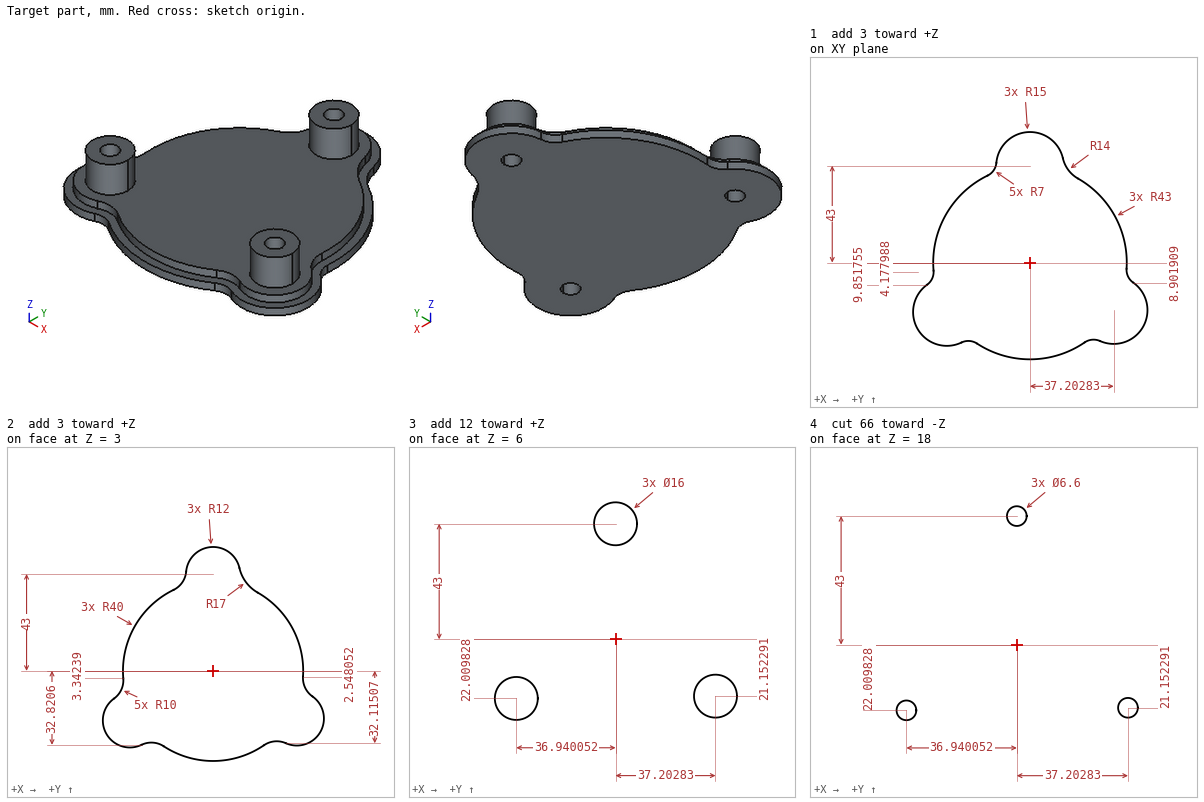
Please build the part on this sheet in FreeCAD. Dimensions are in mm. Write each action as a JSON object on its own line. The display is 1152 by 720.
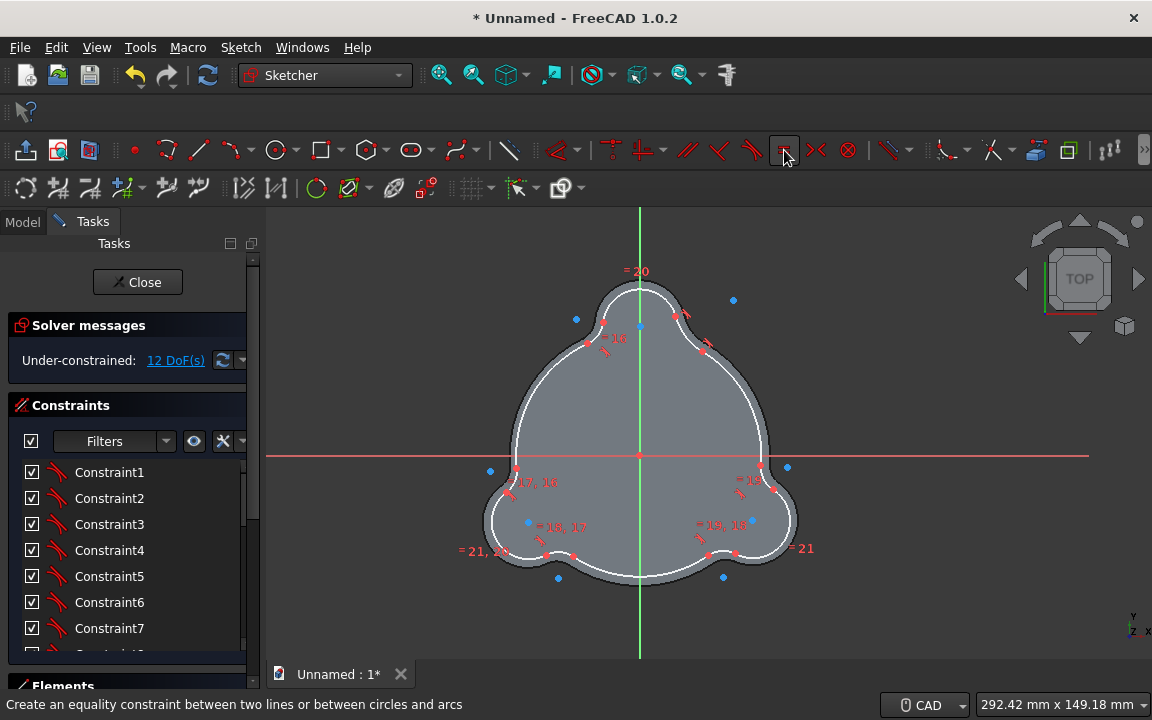
{"action": "left_click", "coordinate": [551, 370]}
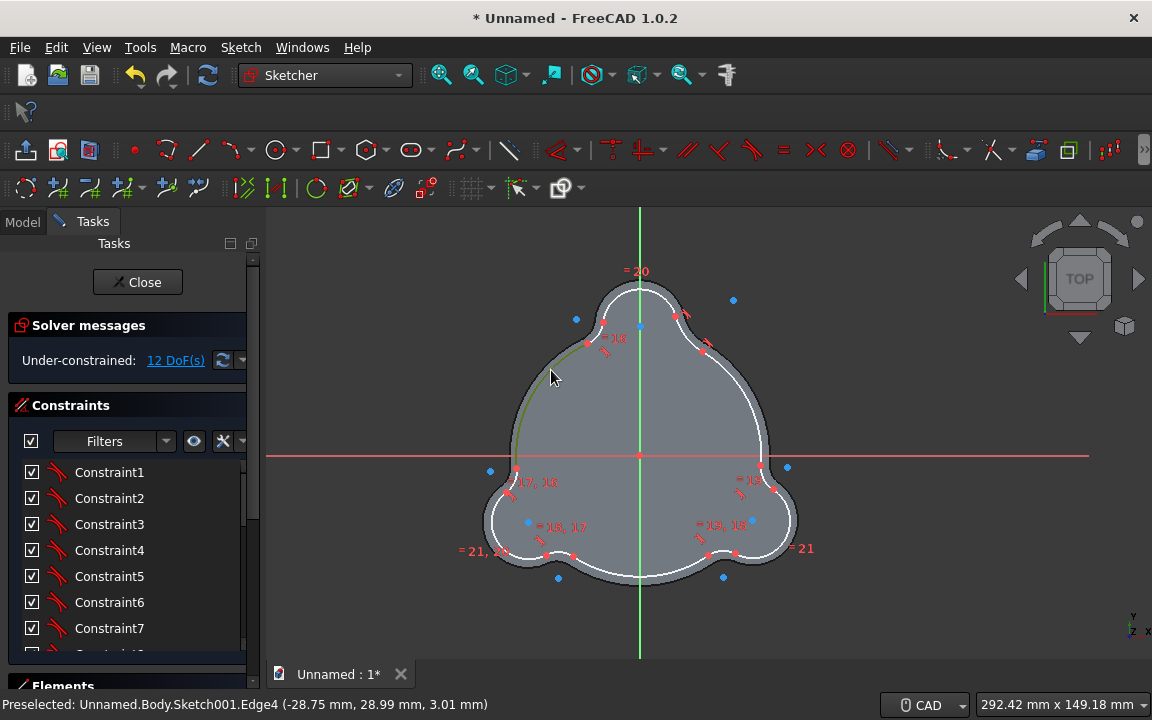
{"action": "left_click", "coordinate": [612, 574]}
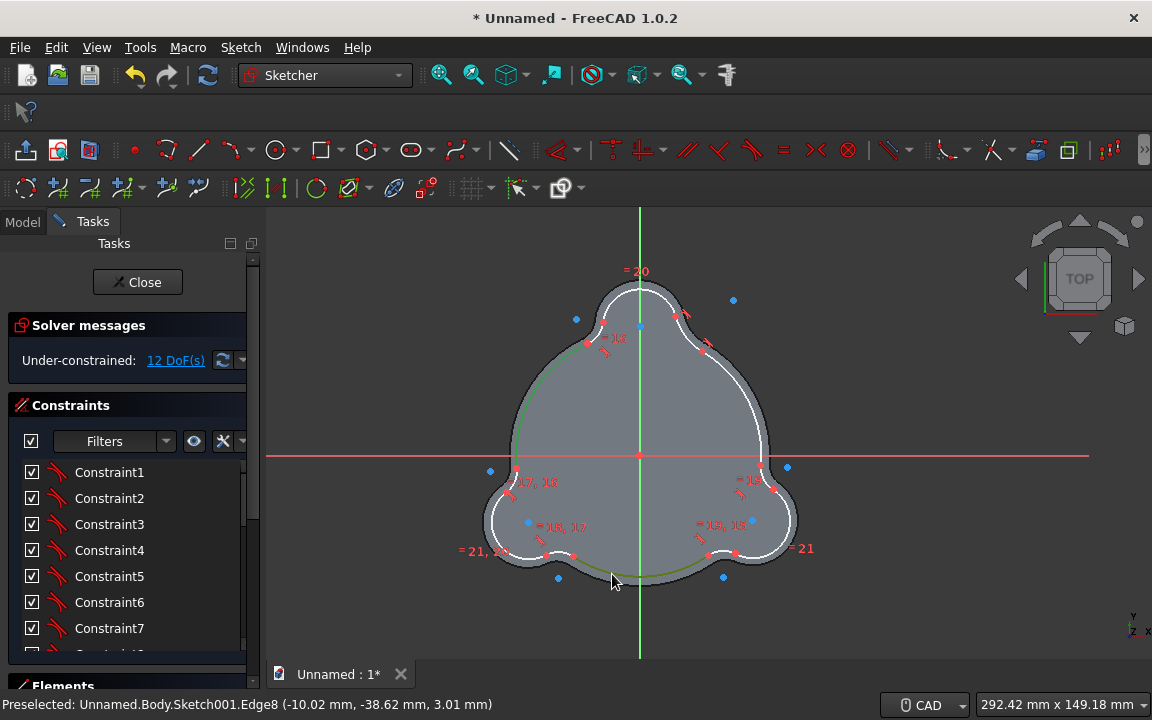
{"action": "left_click", "coordinate": [757, 425]}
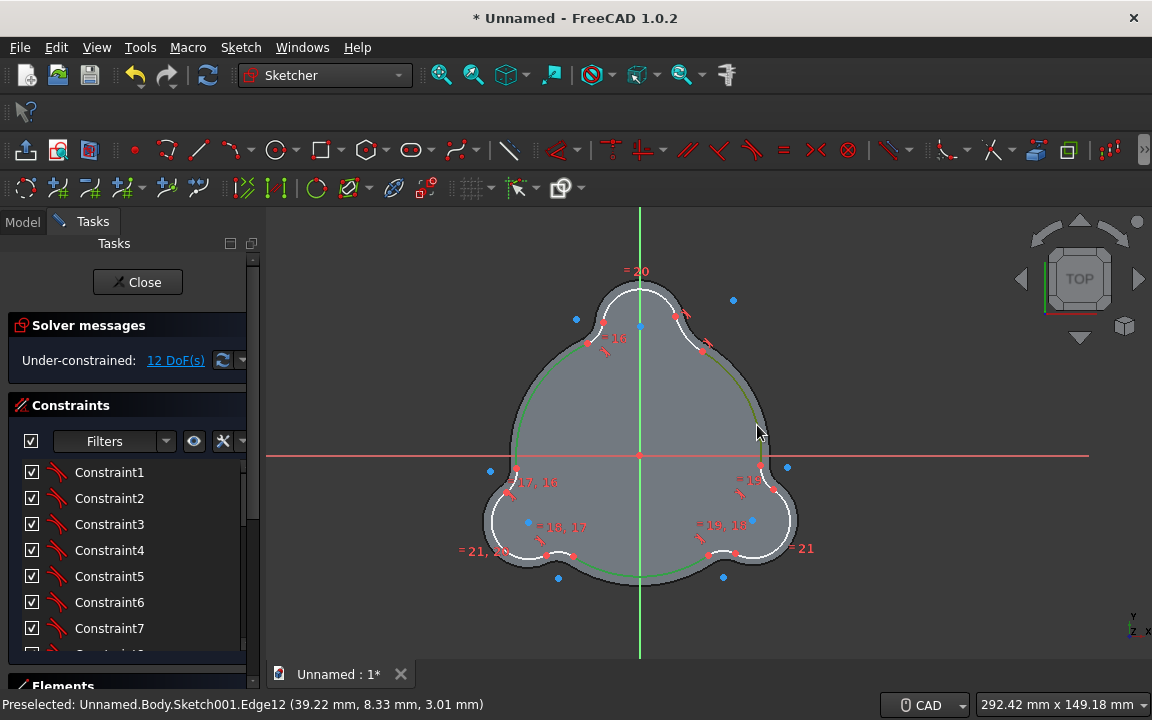
{"action": "left_click", "coordinate": [784, 150]}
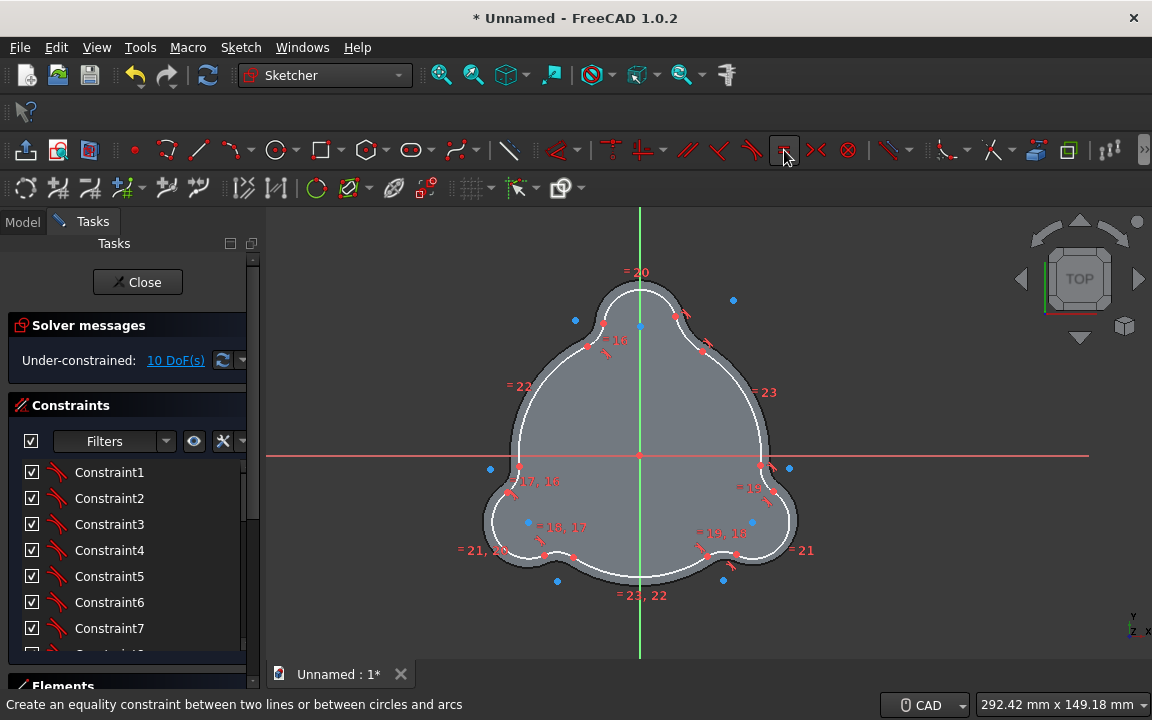
{"action": "left_click", "coordinate": [640, 327]}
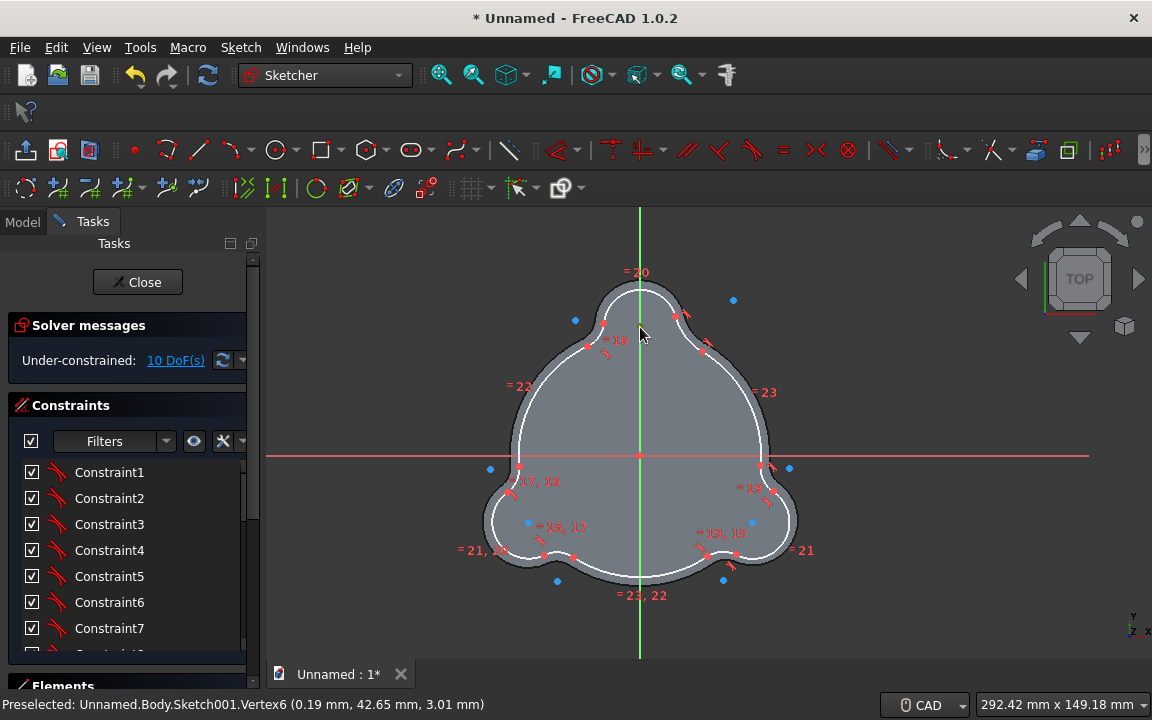
{"action": "left_click", "coordinate": [640, 546]}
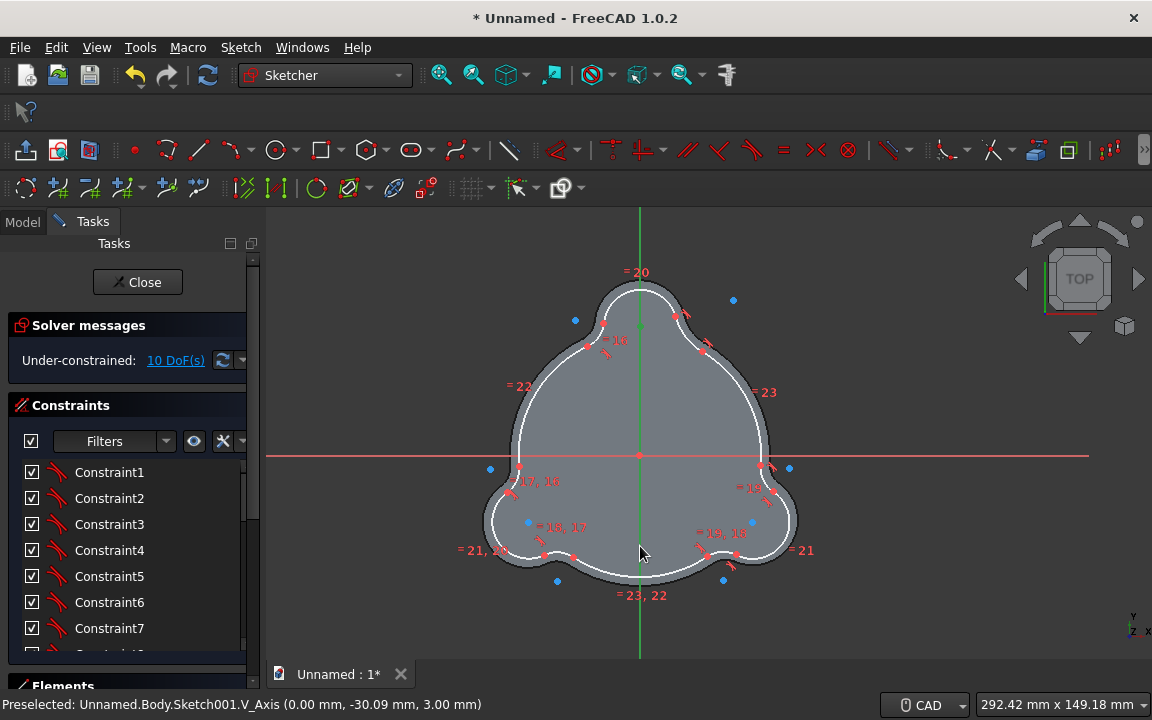
{"action": "left_click", "coordinate": [612, 150]}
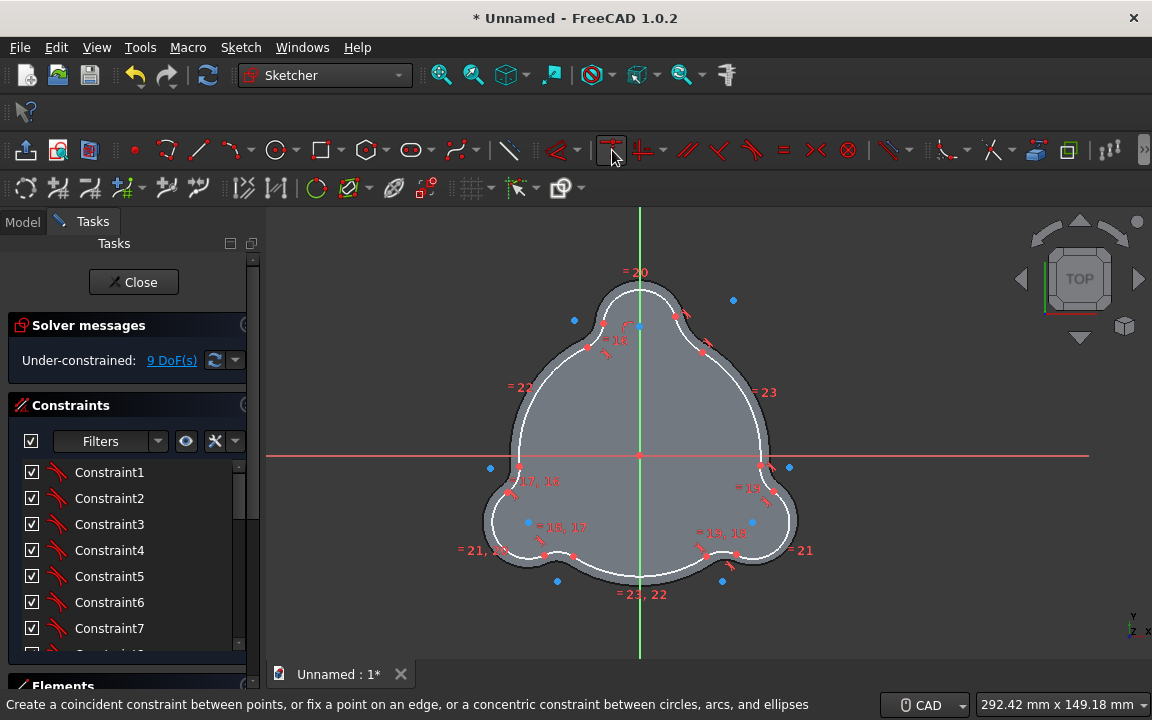
{"action": "left_click", "coordinate": [556, 150]}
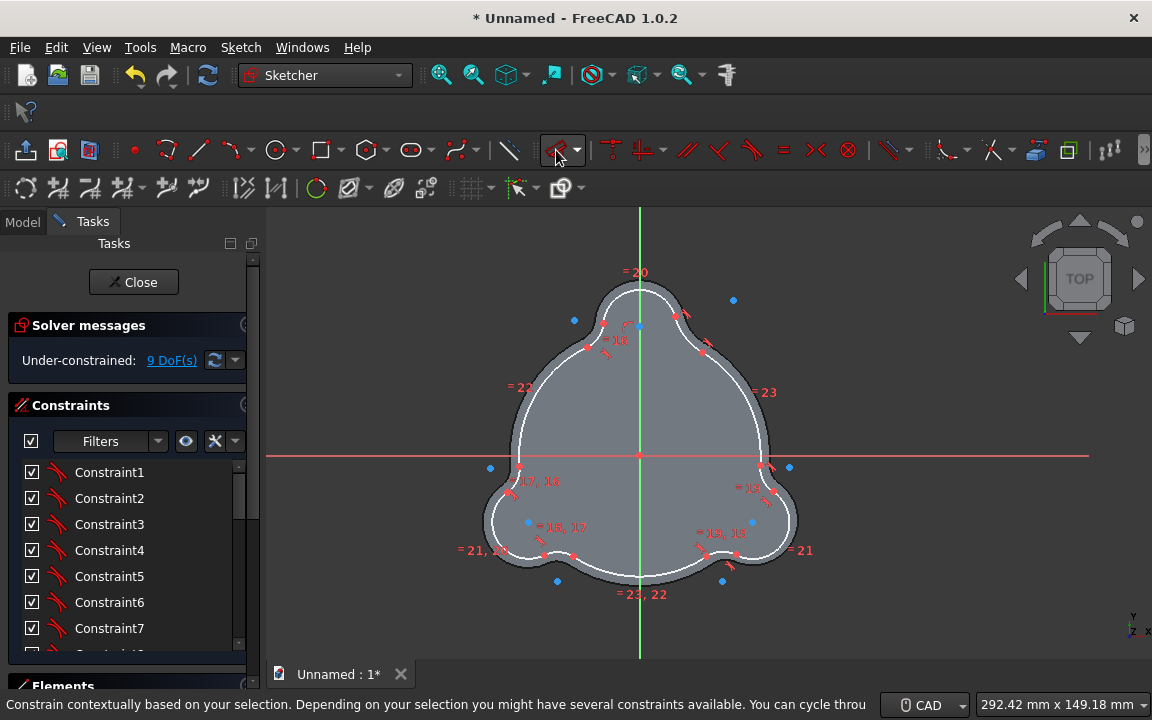
{"action": "left_click", "coordinate": [680, 329]}
{"action": "left_click", "coordinate": [683, 378]}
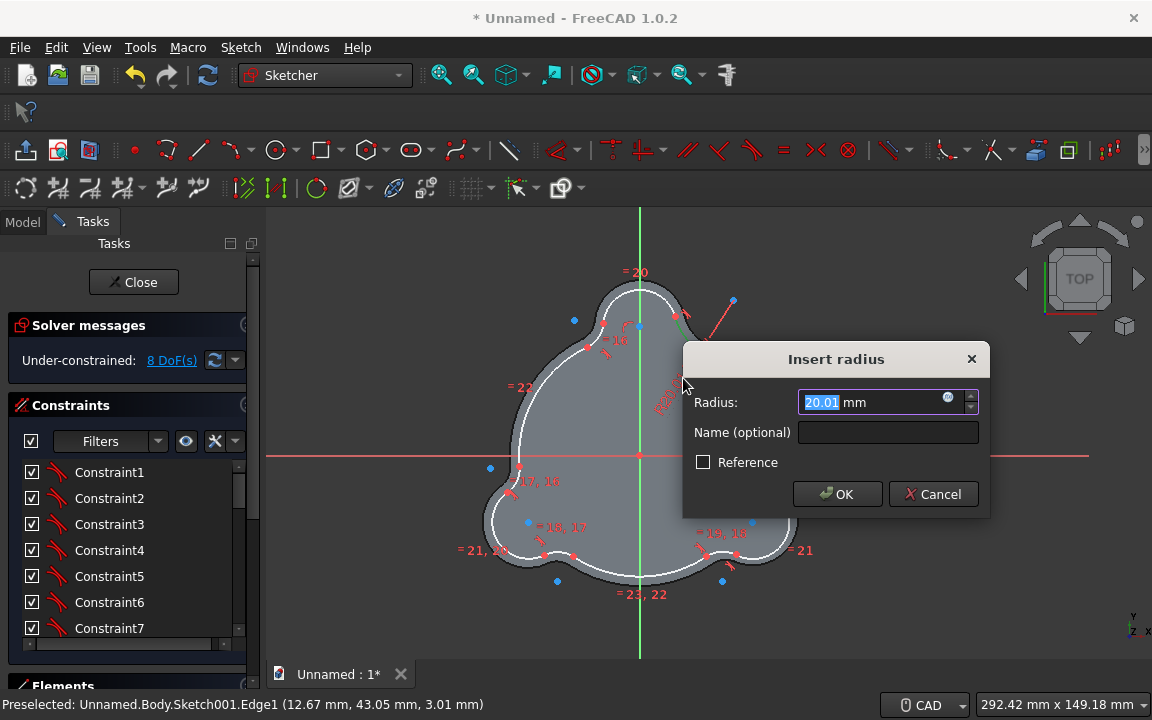
{"action": "type", "text": "17"}
{"action": "key", "text": "Return"}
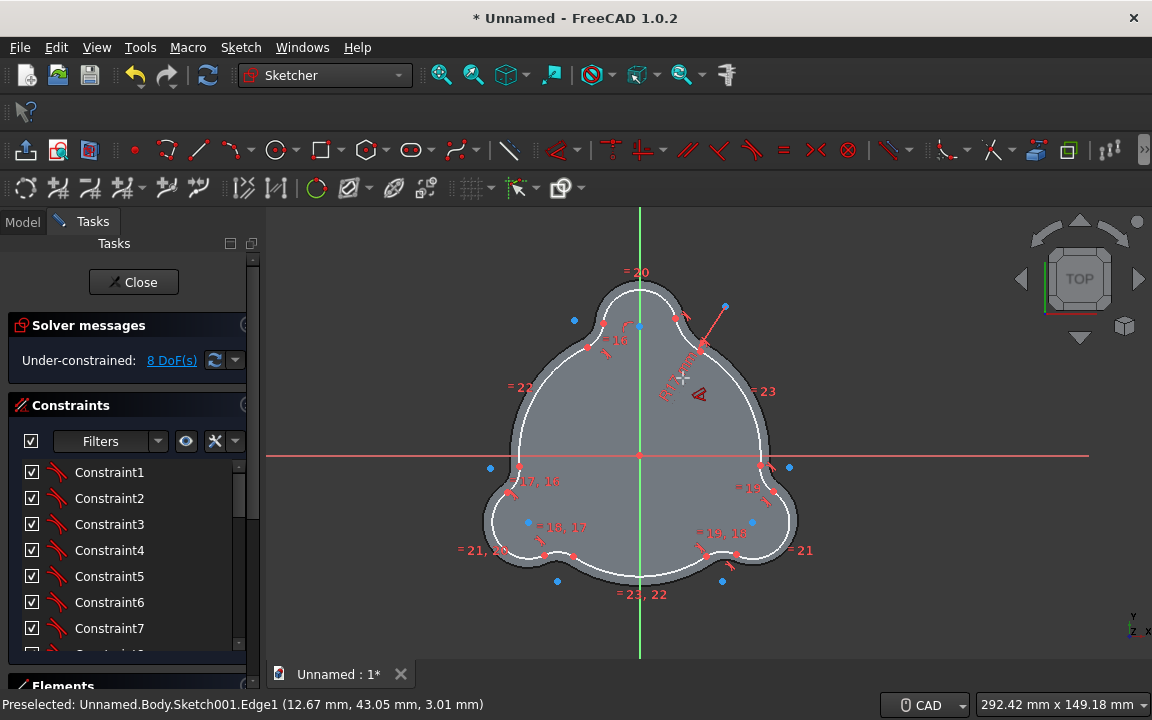
{"action": "left_click", "coordinate": [657, 294]}
{"action": "left_click", "coordinate": [672, 266]}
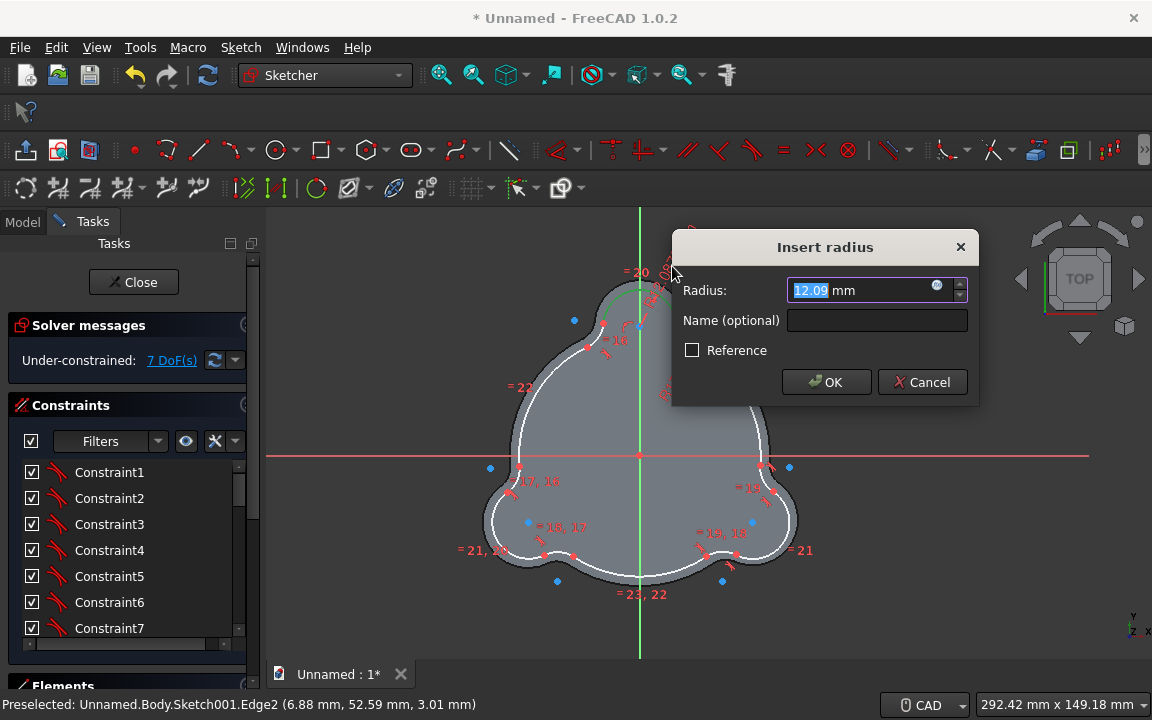
{"action": "type", "text": "12"}
{"action": "key", "text": "Return"}